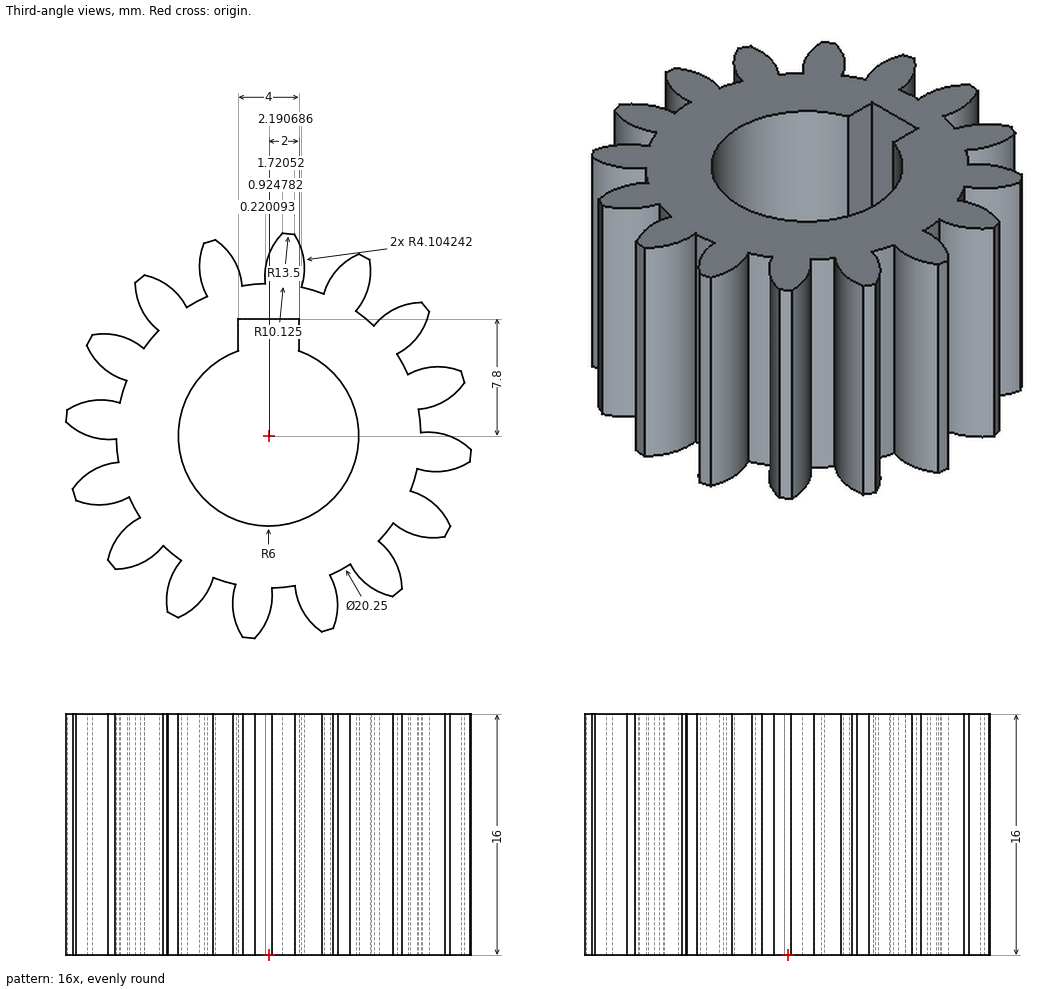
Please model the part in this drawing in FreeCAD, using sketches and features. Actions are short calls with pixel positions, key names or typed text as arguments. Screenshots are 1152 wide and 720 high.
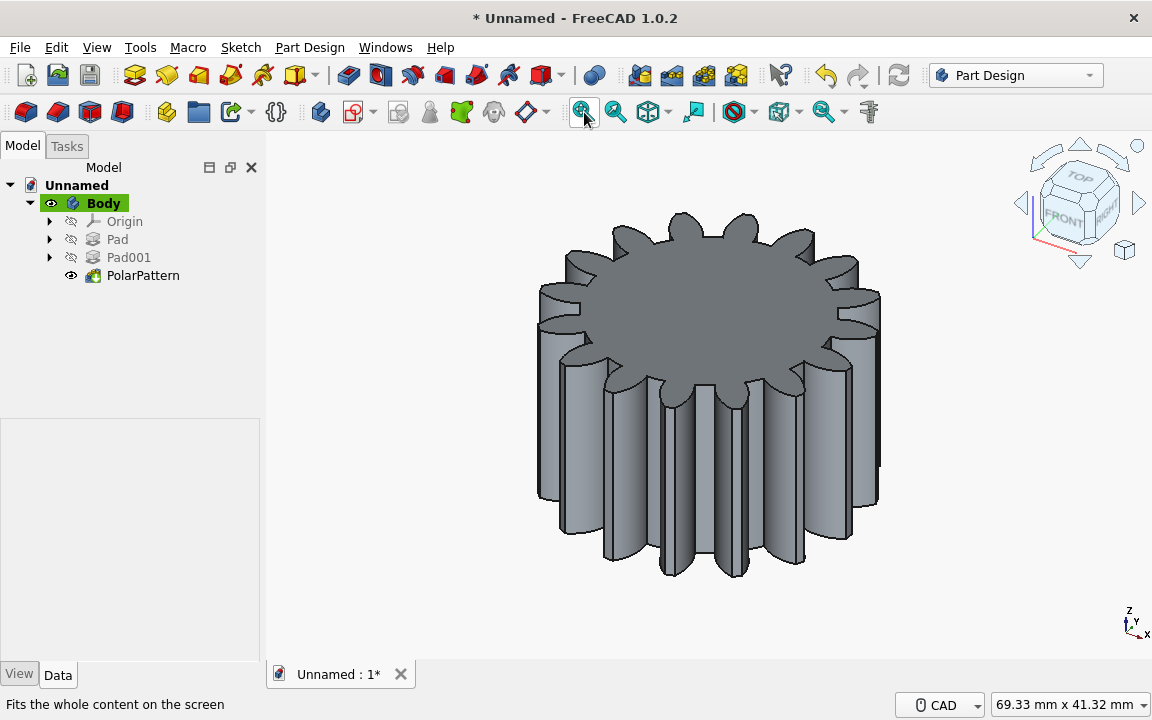
click(709, 310)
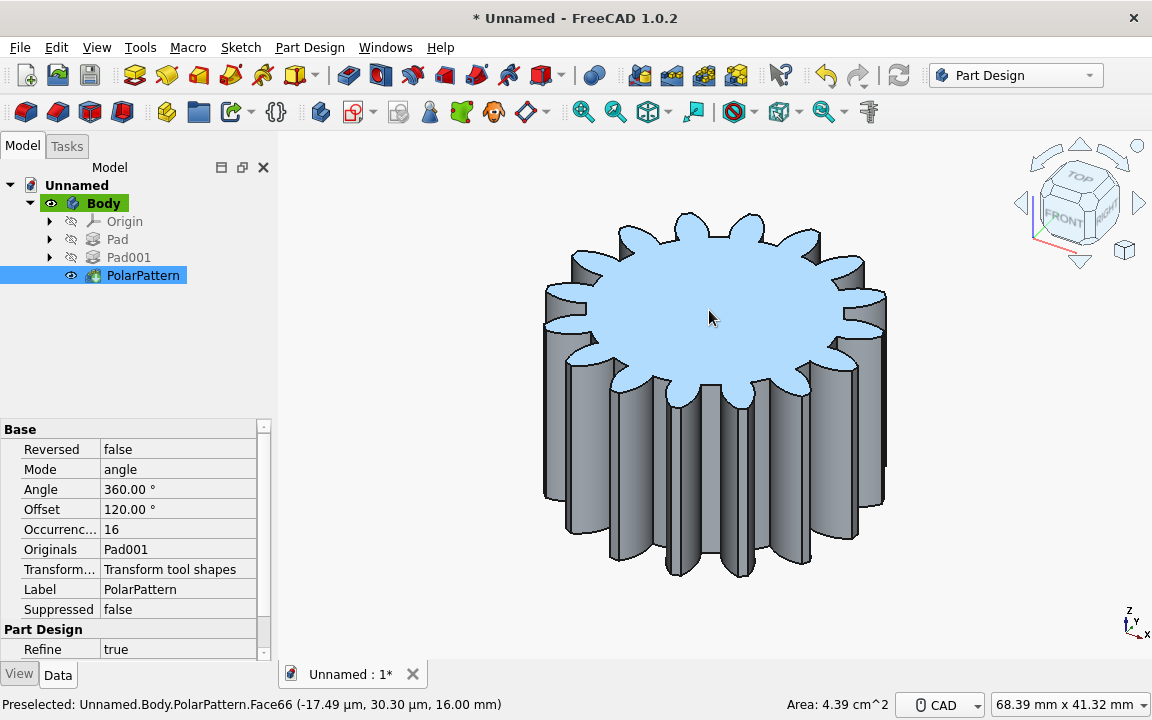
click(354, 112)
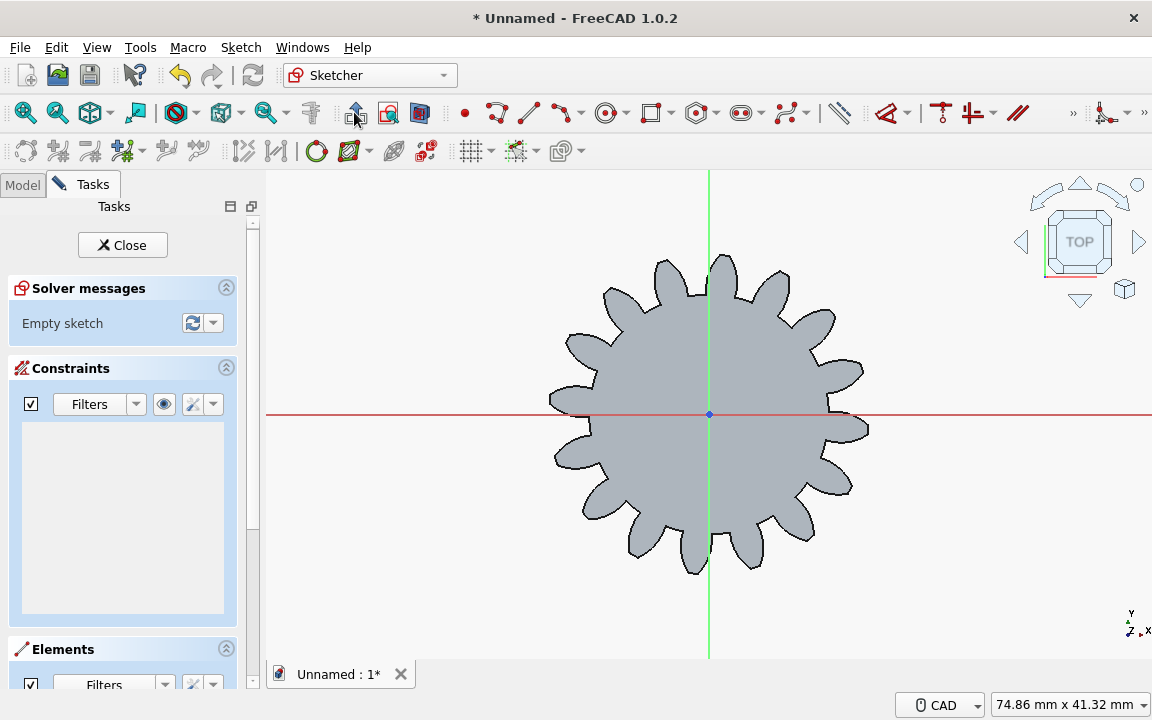
scroll(792, 391, up, 3)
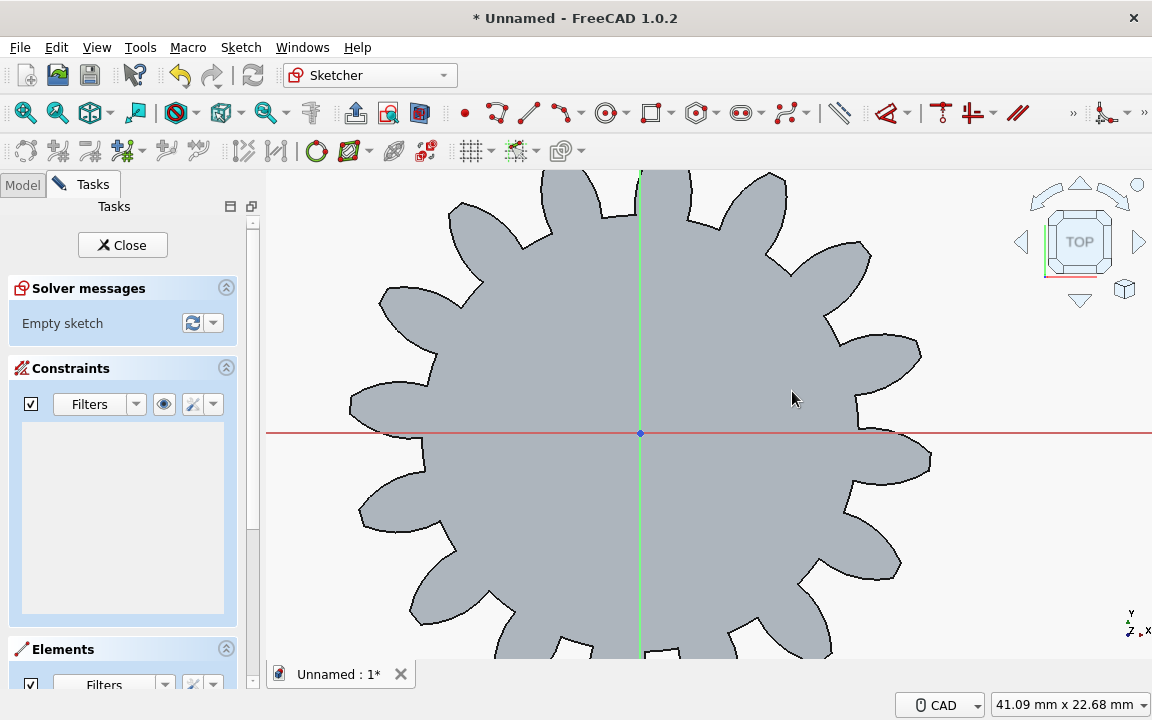
click(498, 114)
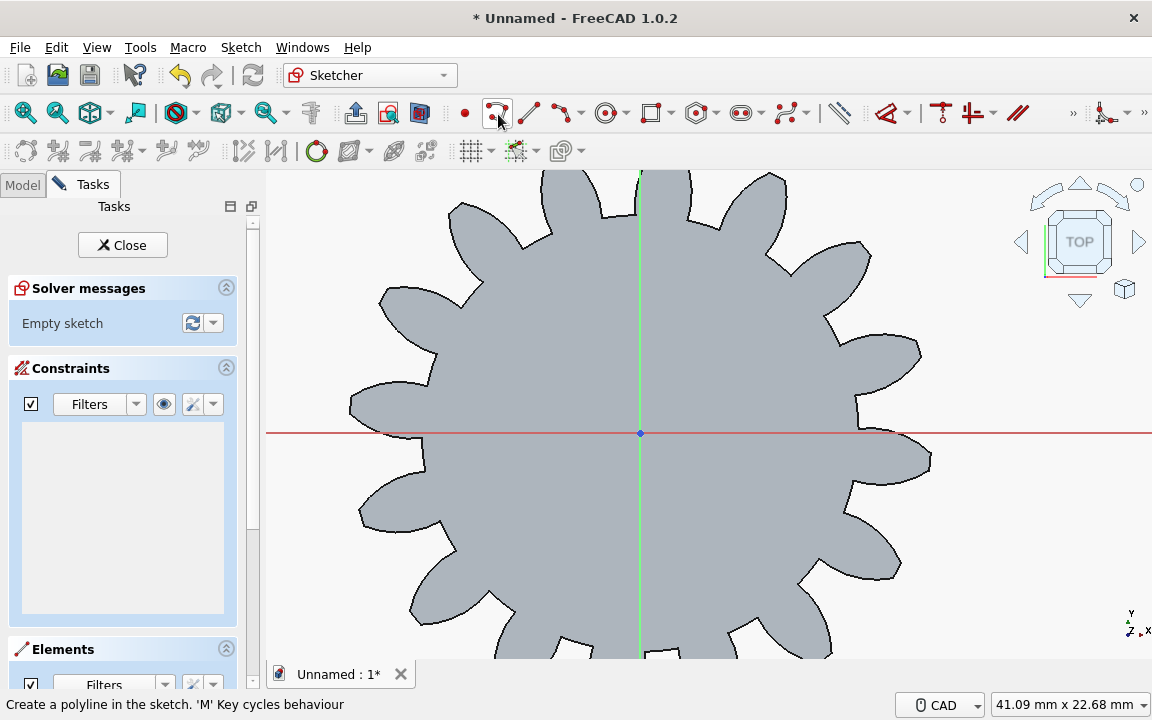
click(683, 311)
click(683, 265)
click(597, 265)
click(597, 311)
right_click(597, 311)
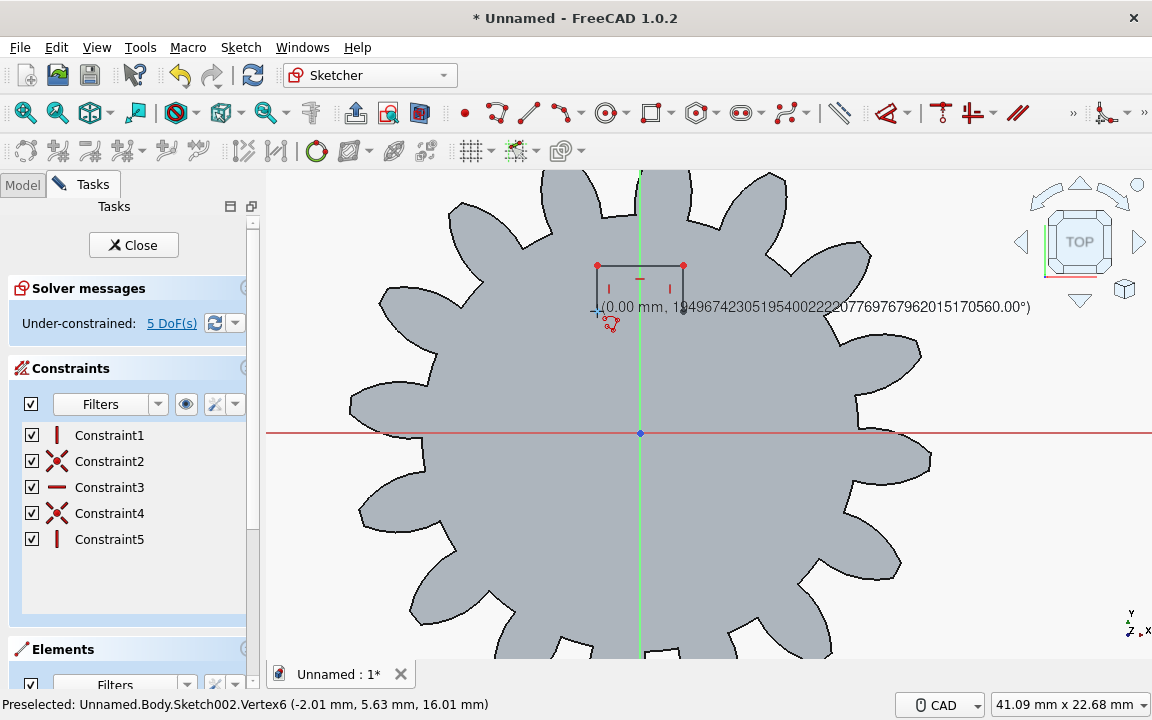
click(562, 114)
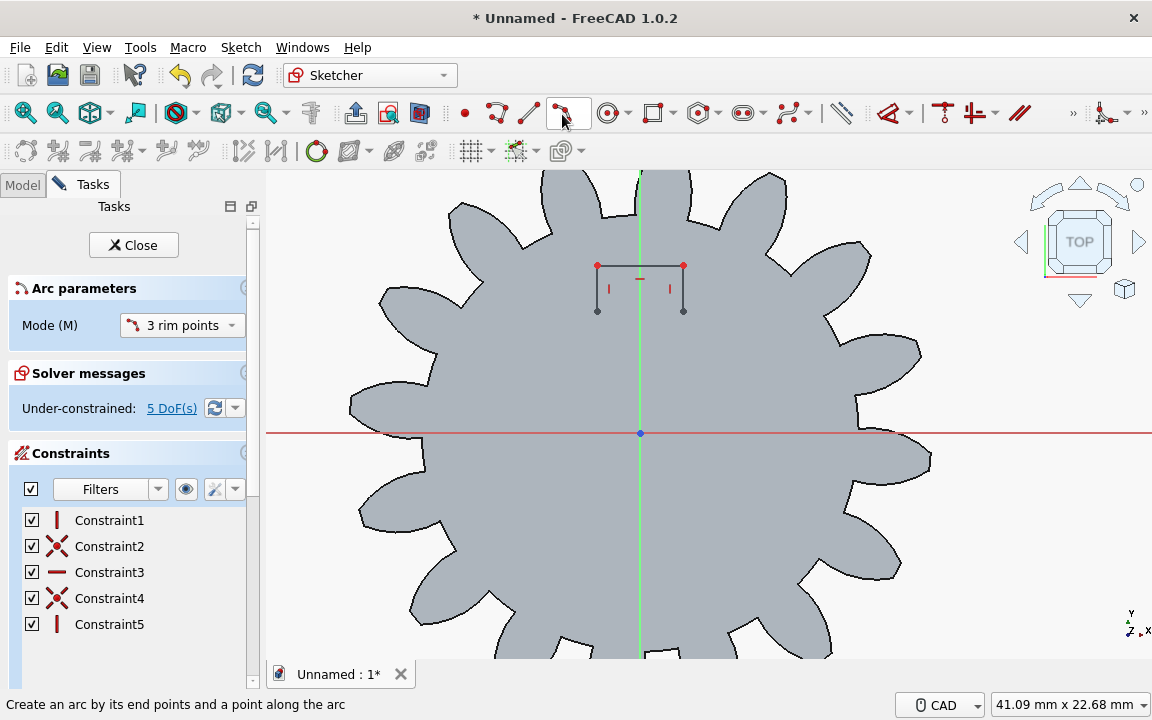
click(597, 312)
click(683, 312)
click(572, 543)
key(Escape)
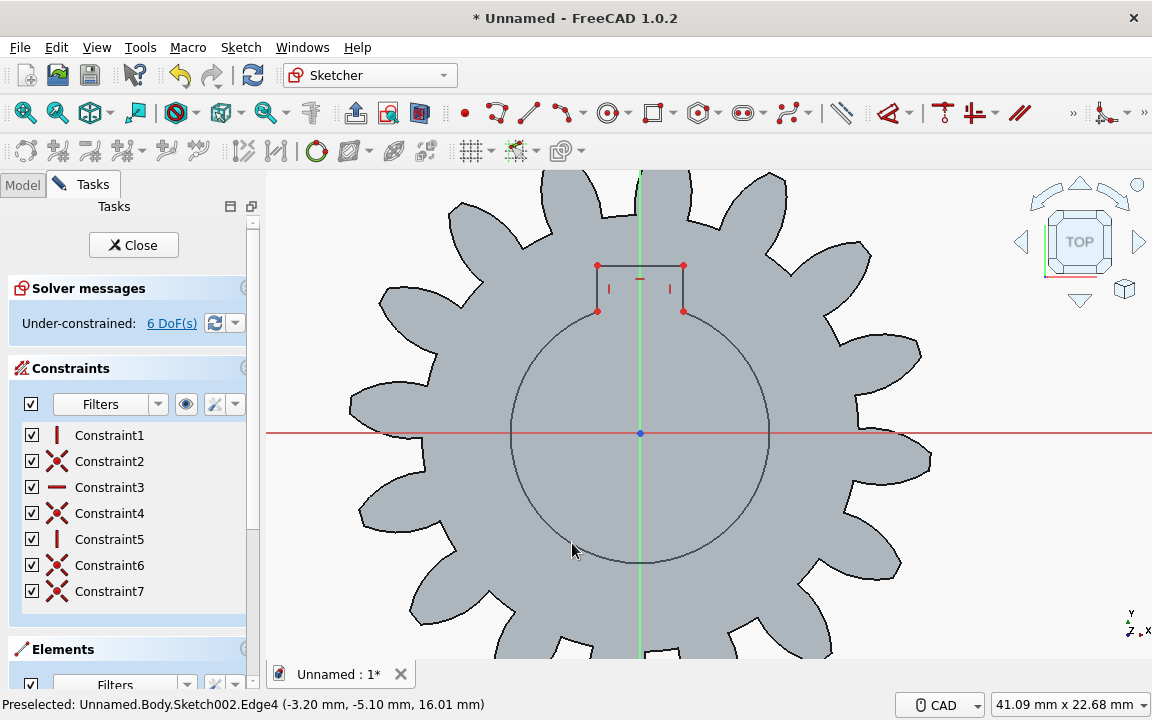
drag(630, 423, 650, 444)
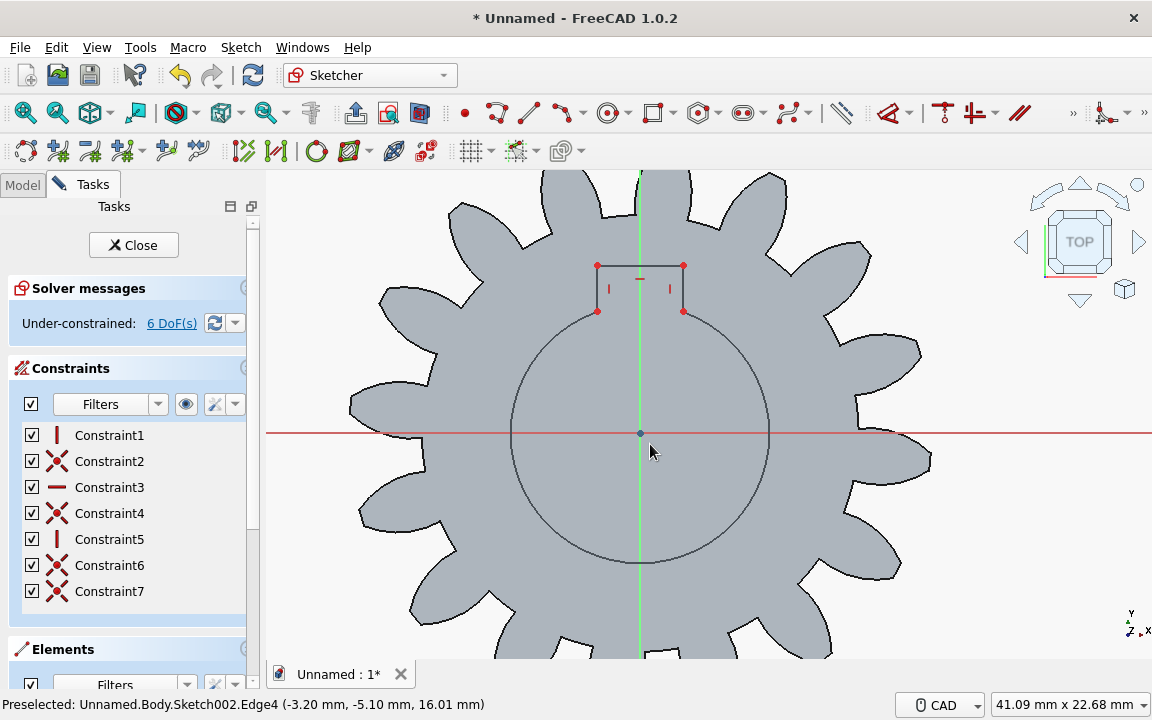
click(944, 114)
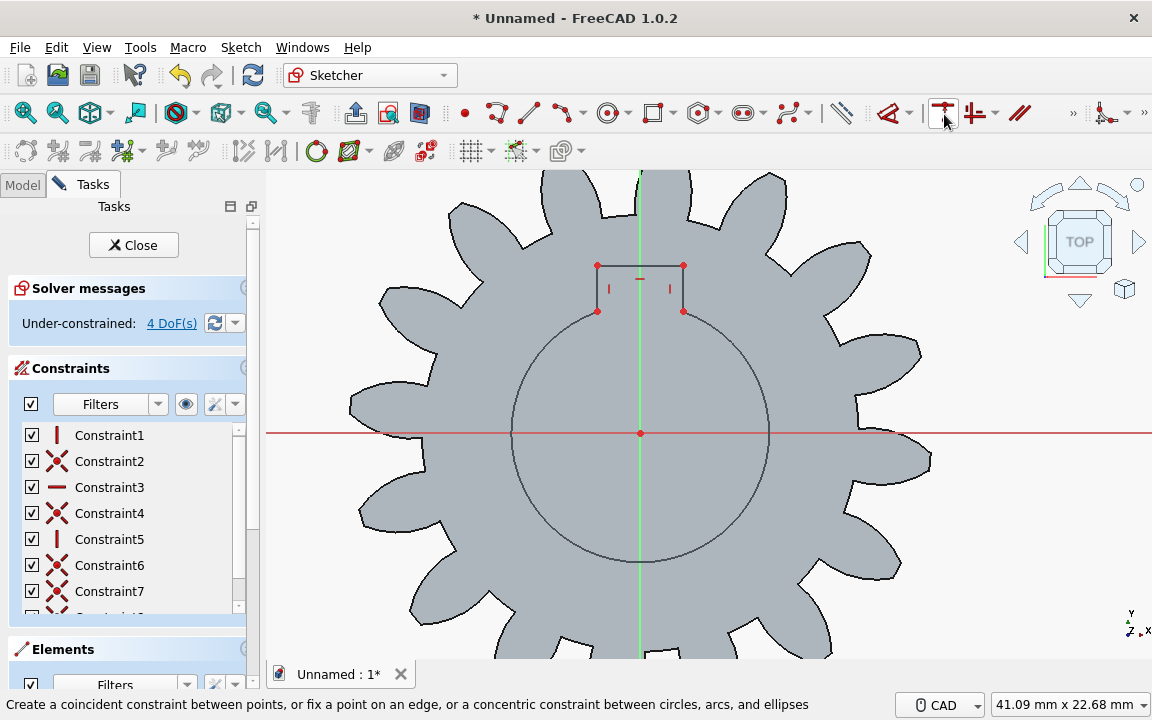
click(888, 114)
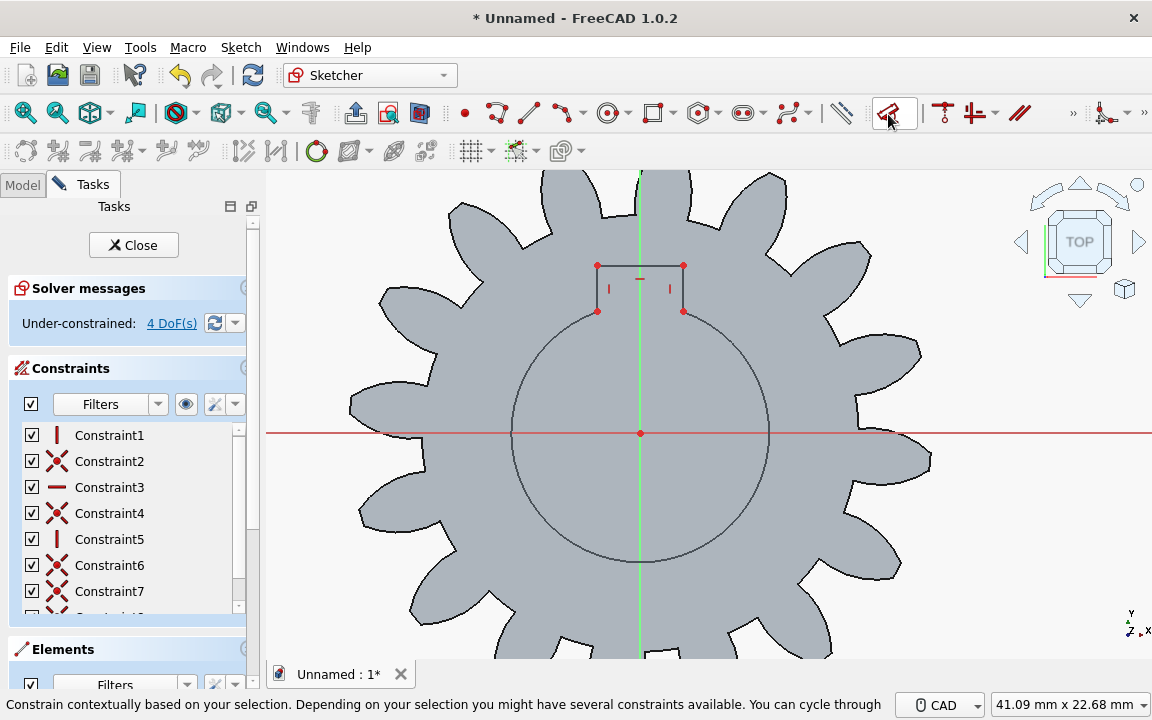
click(524, 490)
click(495, 504)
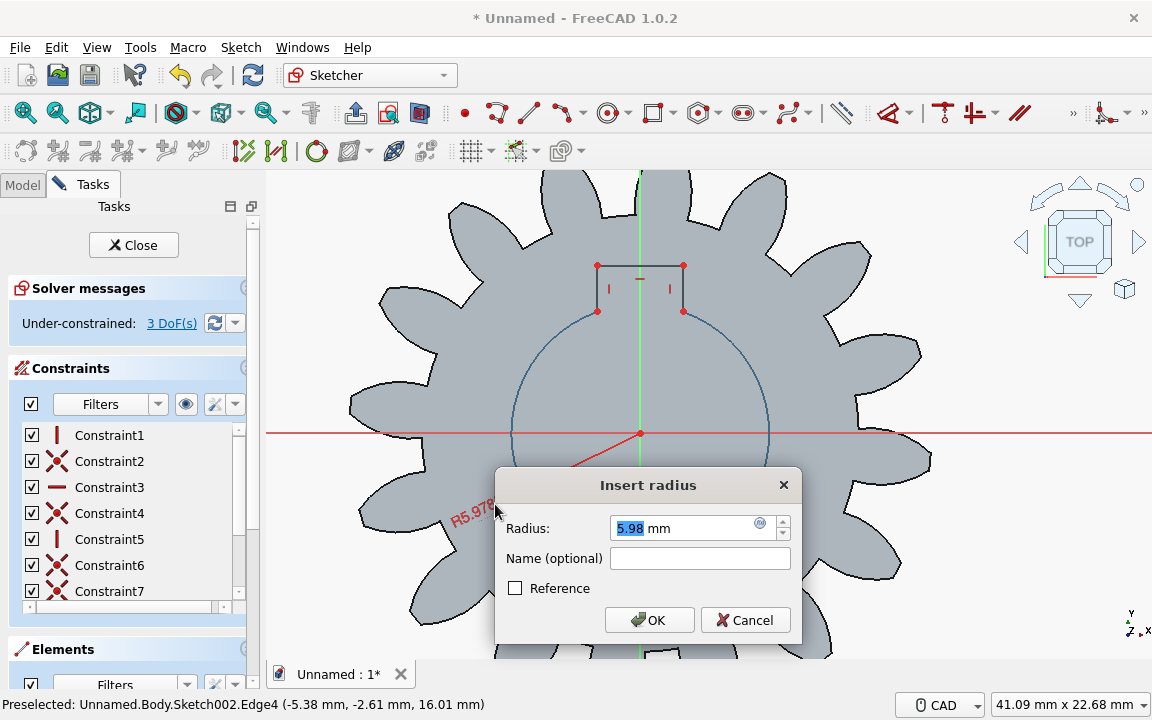
text(6)
key(Return)